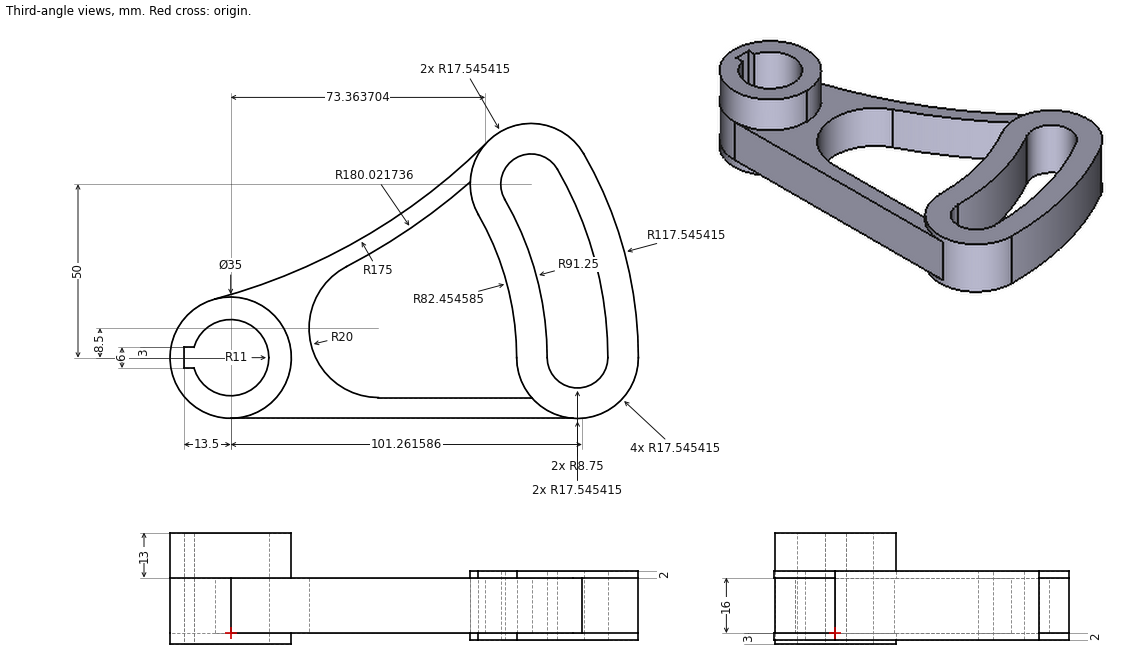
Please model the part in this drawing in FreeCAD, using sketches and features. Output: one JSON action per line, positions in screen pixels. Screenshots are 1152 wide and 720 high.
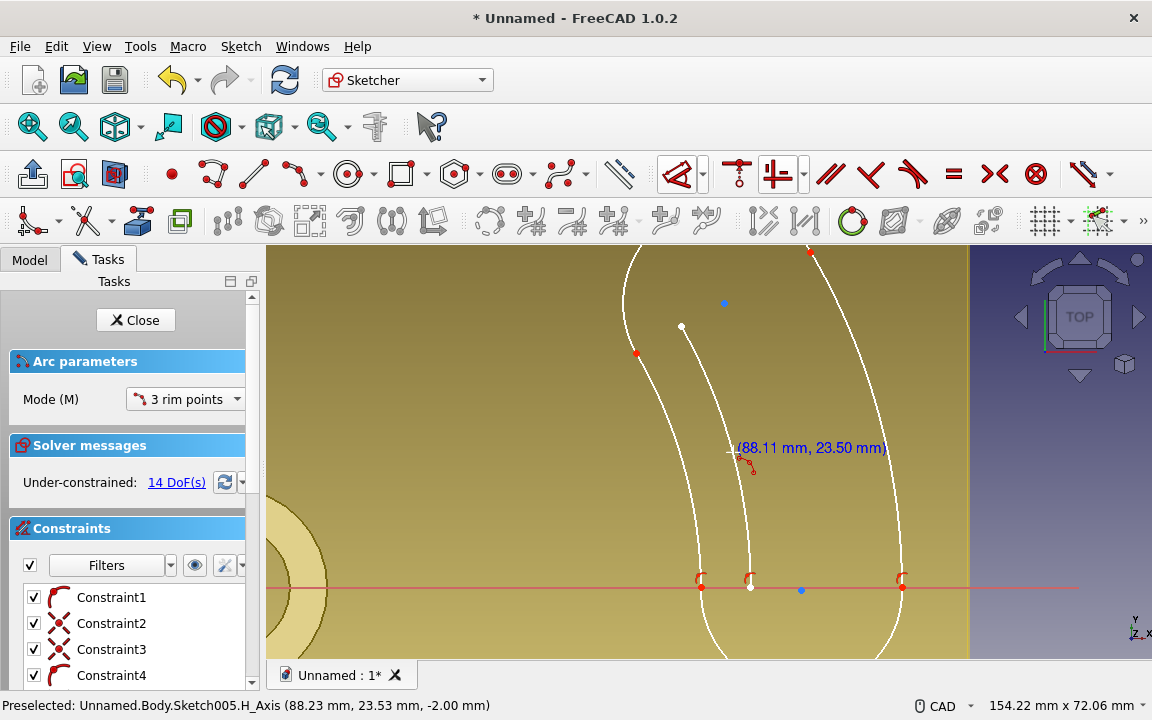
{"action": "left_click", "coordinate": [751, 588]}
{"action": "left_click", "coordinate": [852, 588]}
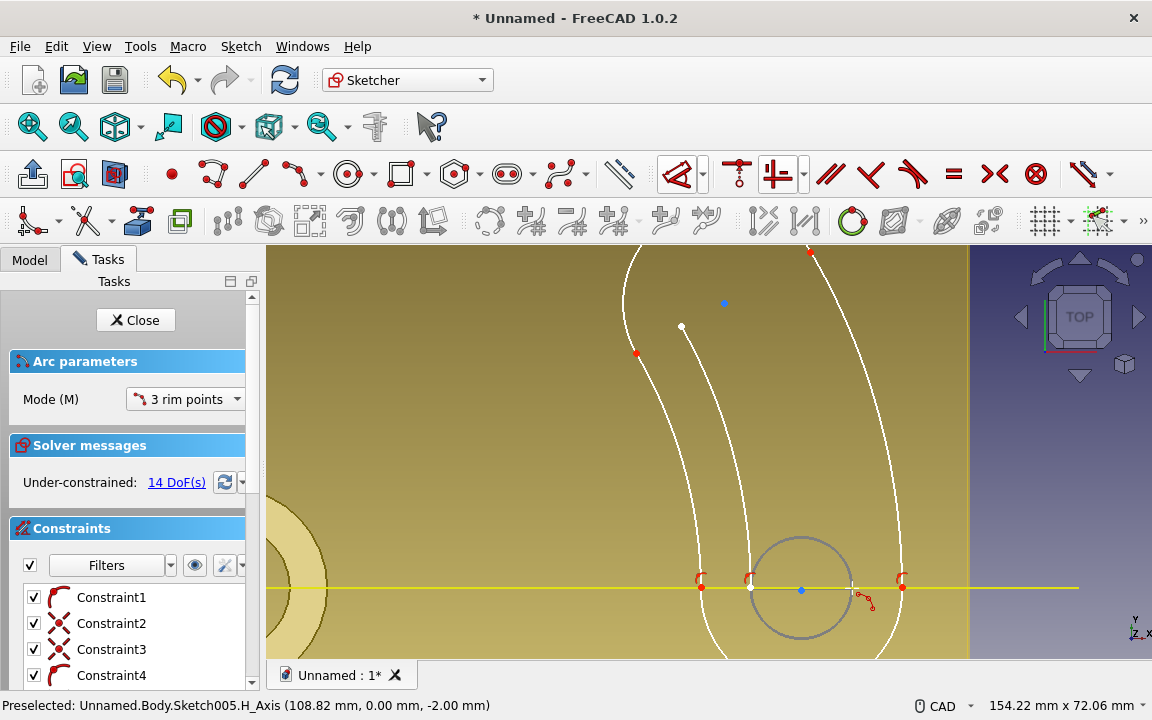
{"action": "scroll", "coordinate": [733, 453], "scroll_direction": "down", "scroll_amount": 3}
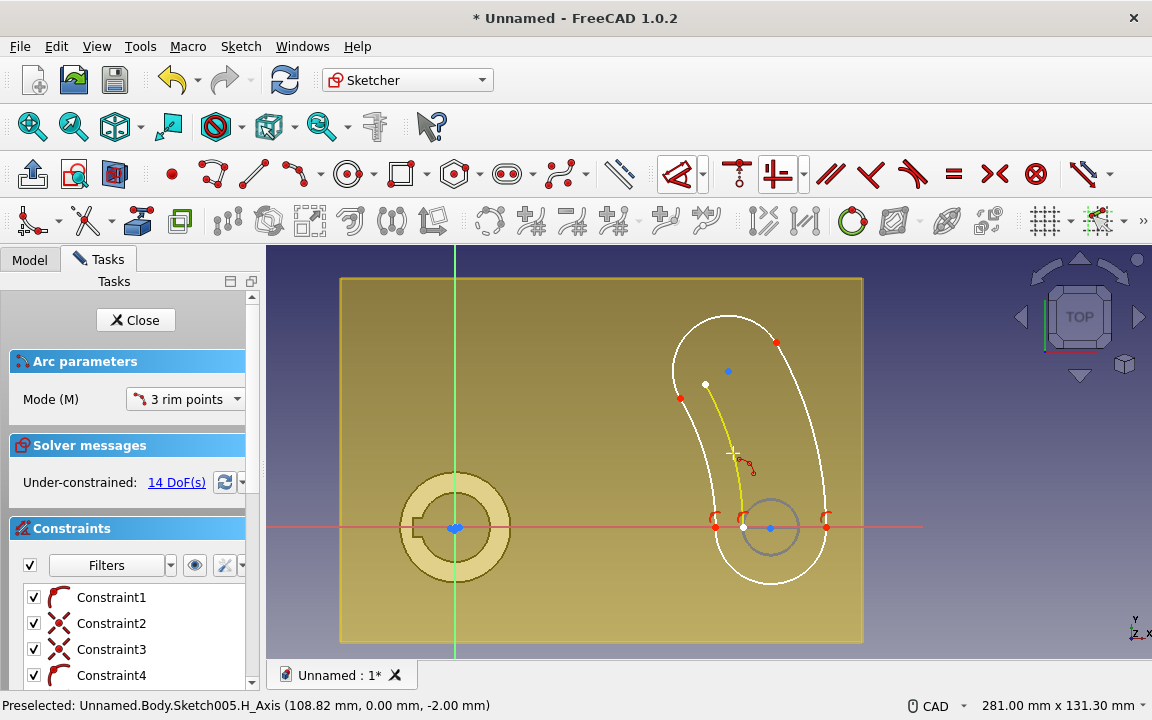
{"action": "left_click", "coordinate": [771, 555]}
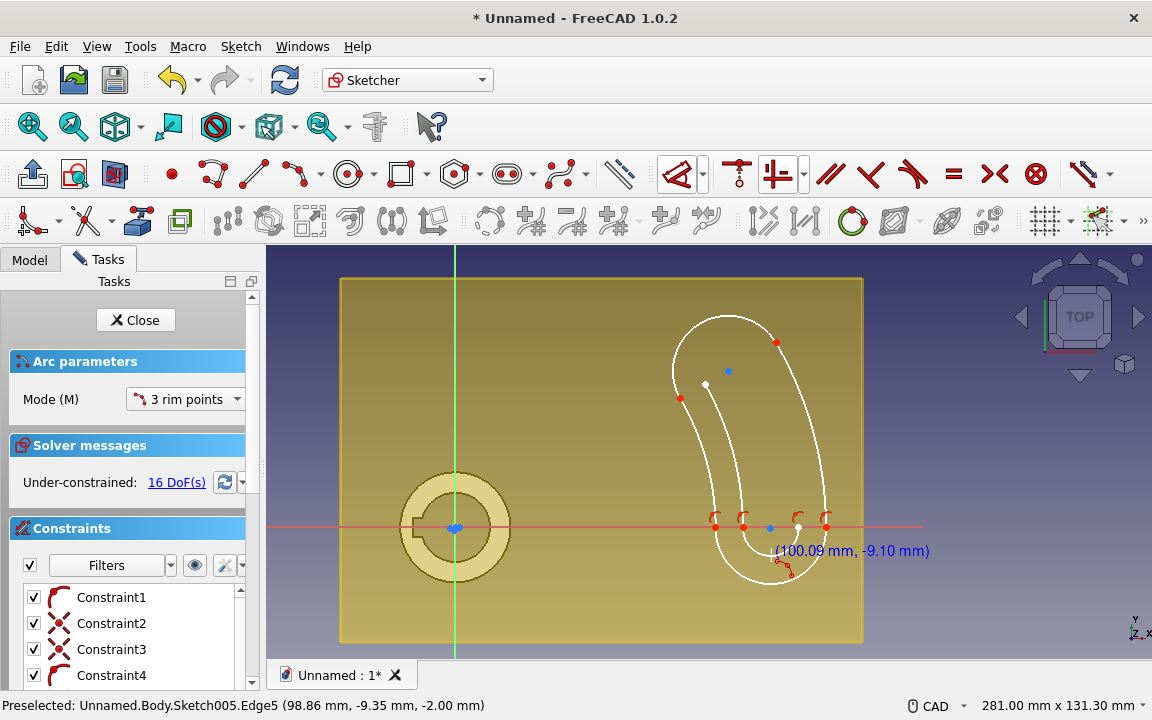
{"action": "left_click", "coordinate": [799, 527]}
{"action": "left_click", "coordinate": [752, 356]}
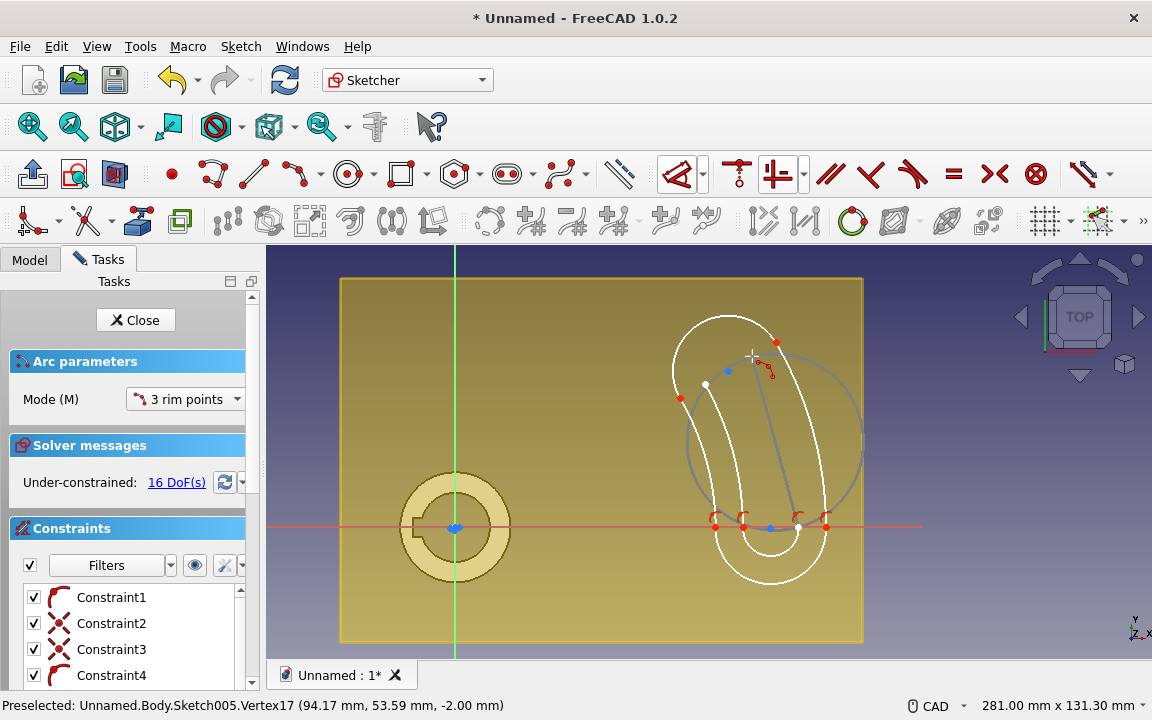
{"action": "scroll", "coordinate": [787, 439], "scroll_direction": "up", "scroll_amount": 2}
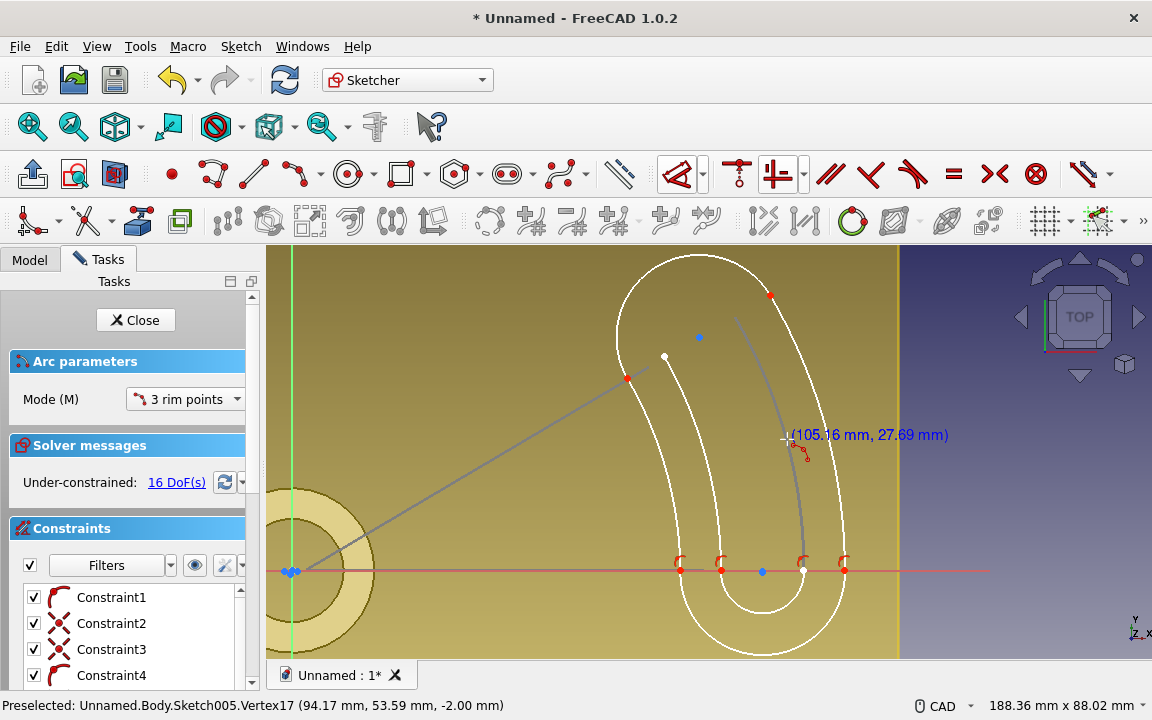
{"action": "left_click", "coordinate": [786, 438]}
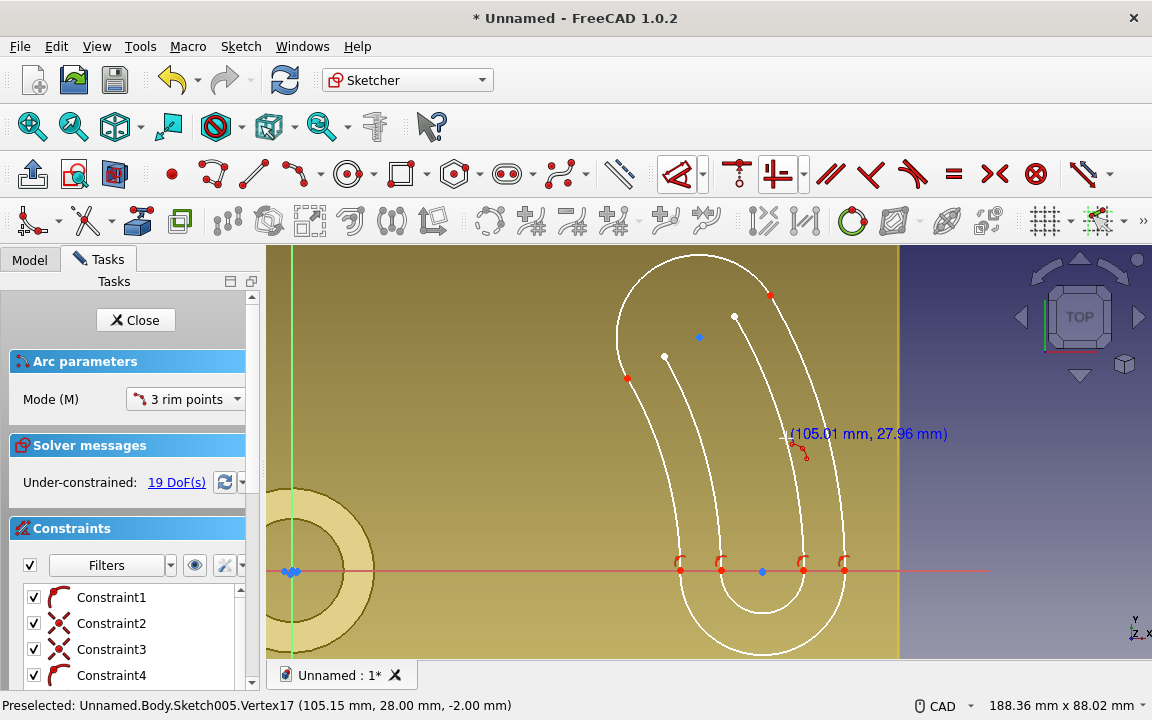
{"action": "left_click", "coordinate": [734, 316]}
{"action": "left_click", "coordinate": [664, 357]}
{"action": "left_click", "coordinate": [679, 300]}
{"action": "key", "text": "Escape"}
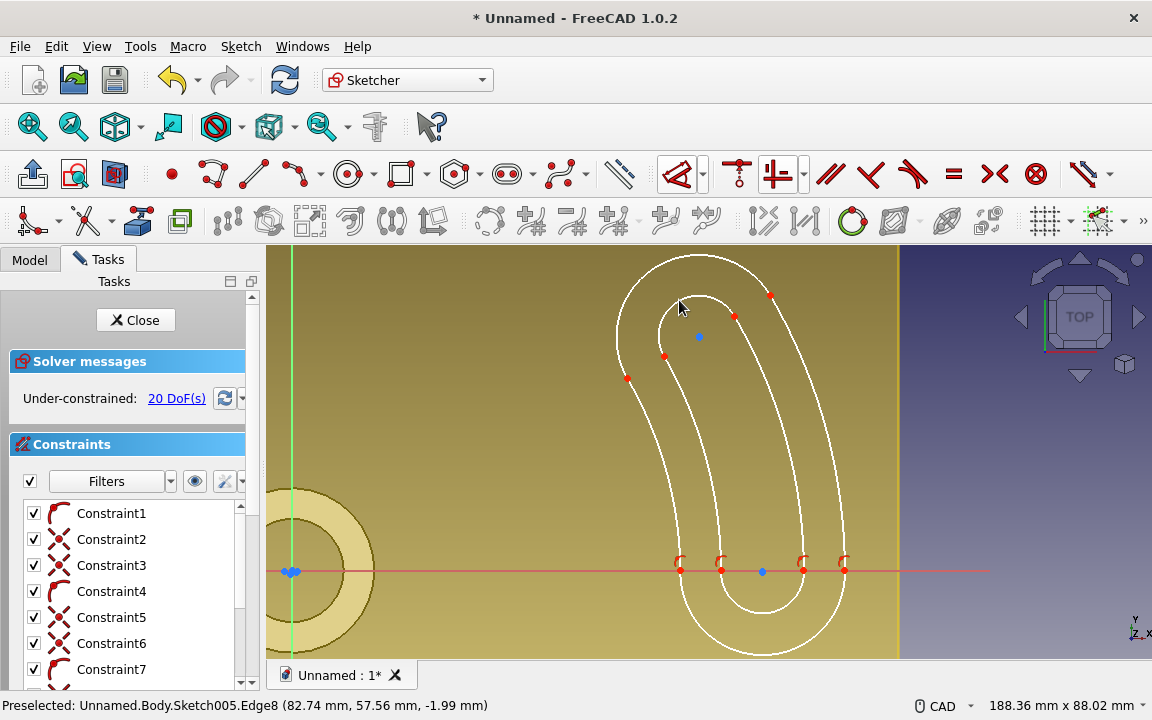
{"action": "left_click", "coordinate": [675, 510]}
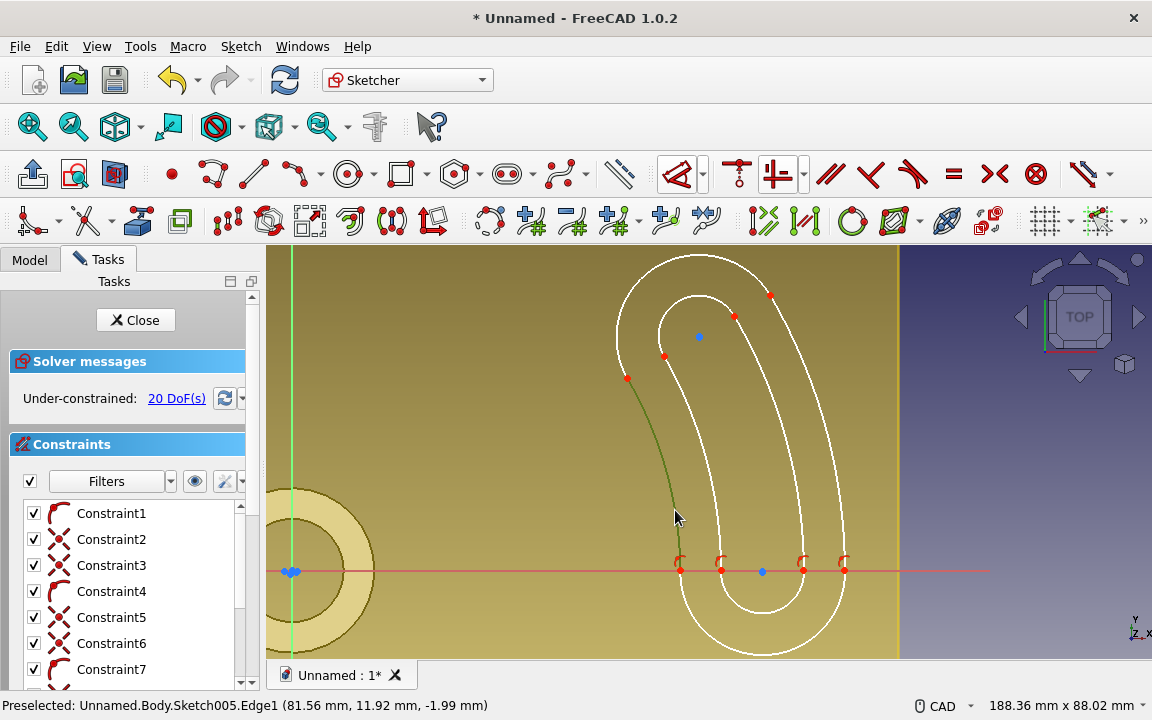
{"action": "left_click", "coordinate": [624, 304]}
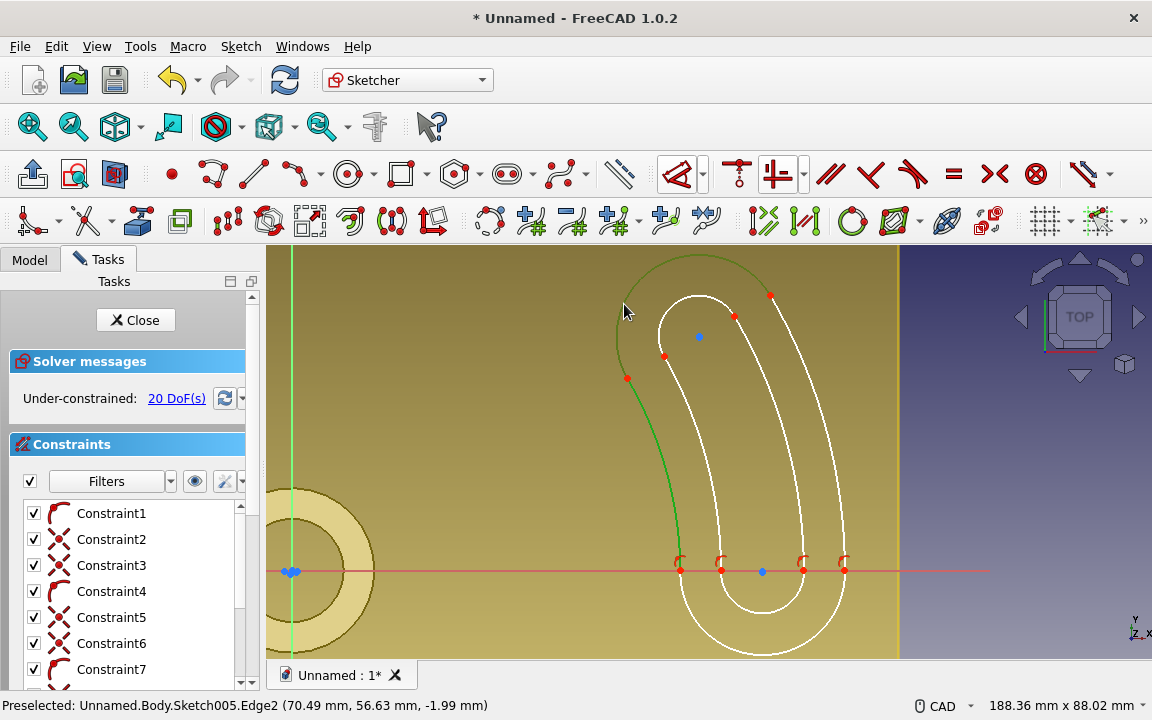
{"action": "left_click", "coordinate": [913, 174]}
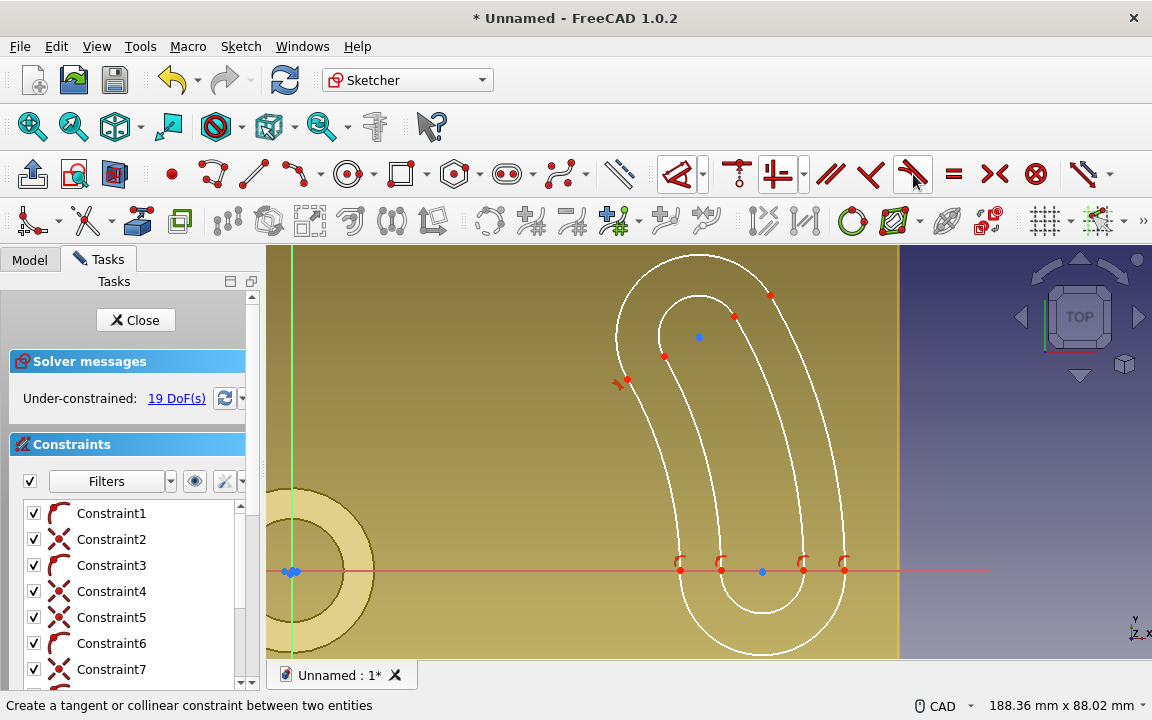
{"action": "left_click", "coordinate": [675, 511]}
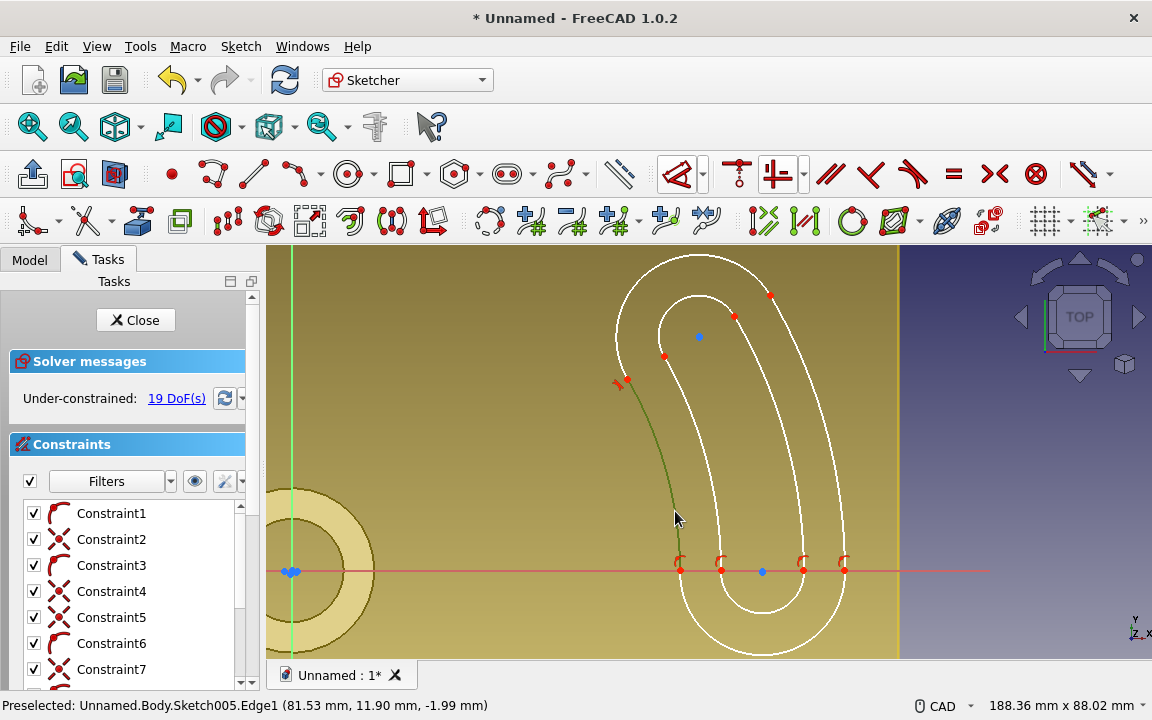
{"action": "left_click", "coordinate": [695, 620]}